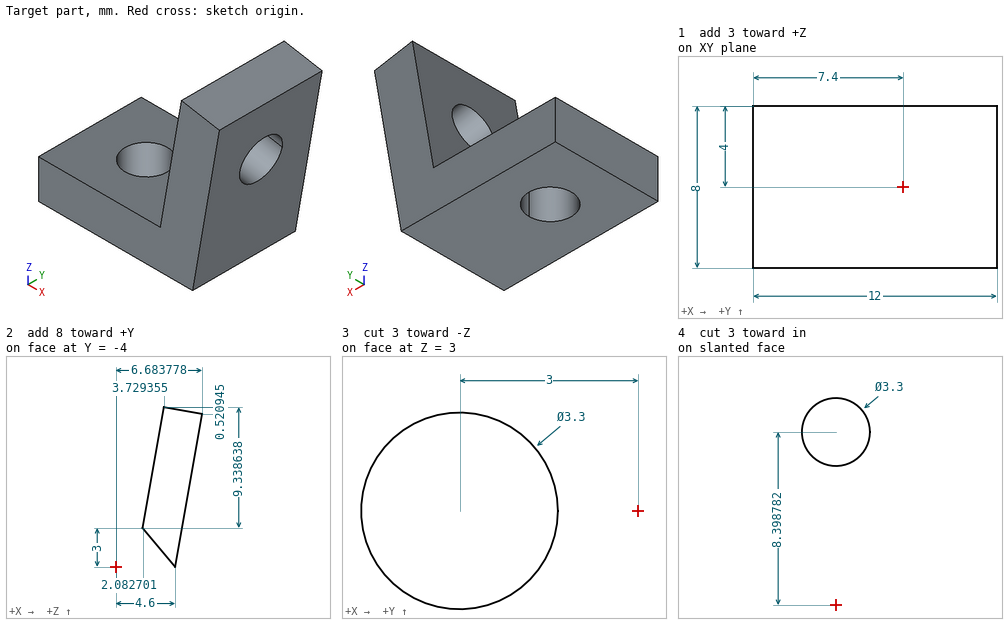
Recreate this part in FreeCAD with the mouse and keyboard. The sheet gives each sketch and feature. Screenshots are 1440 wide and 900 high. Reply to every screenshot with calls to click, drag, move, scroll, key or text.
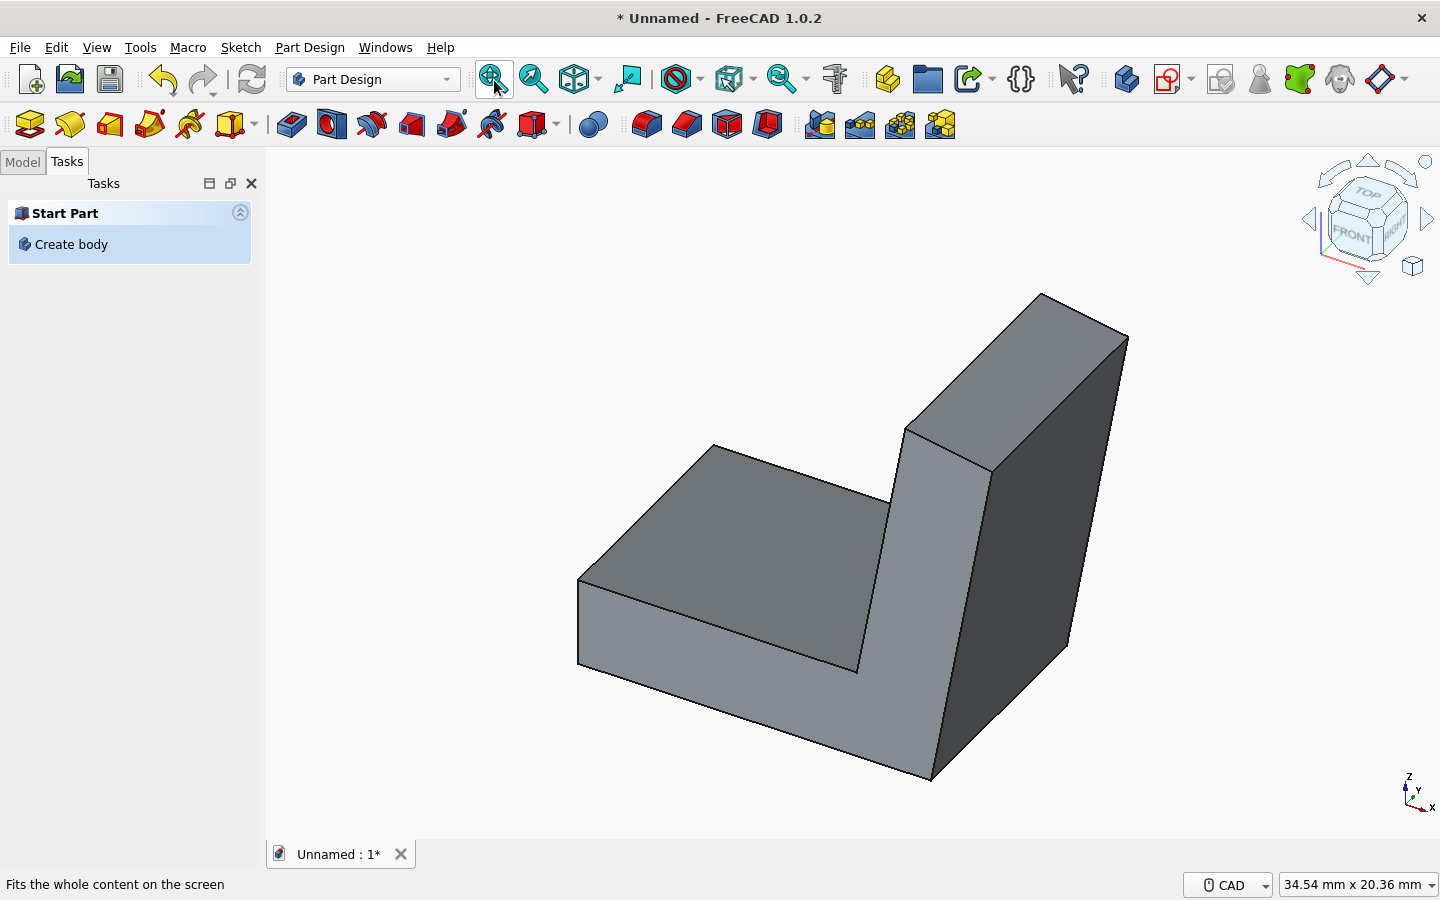
click(785, 558)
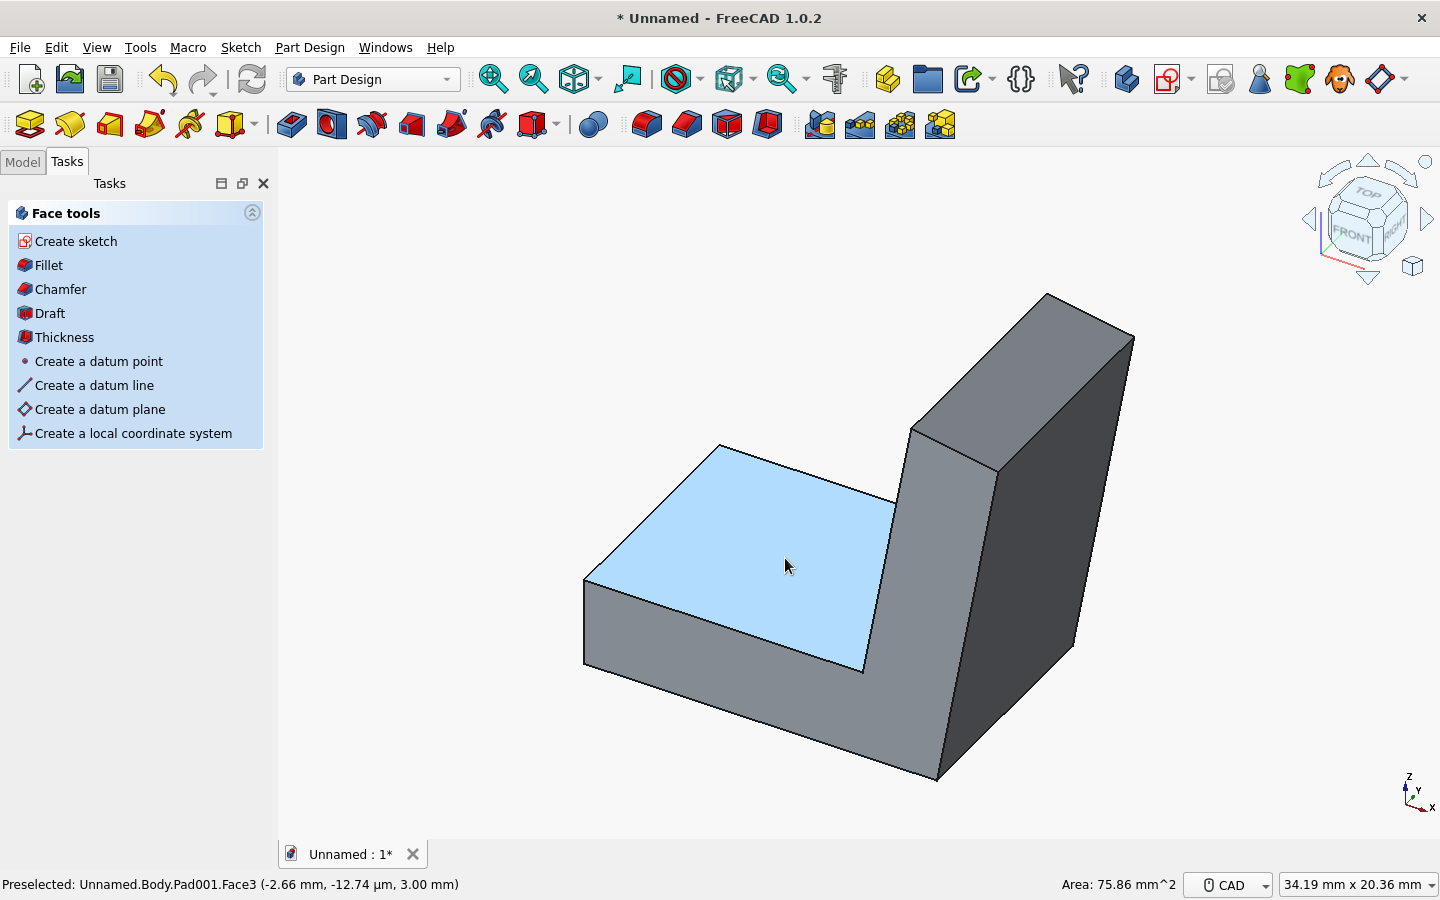
click(1168, 80)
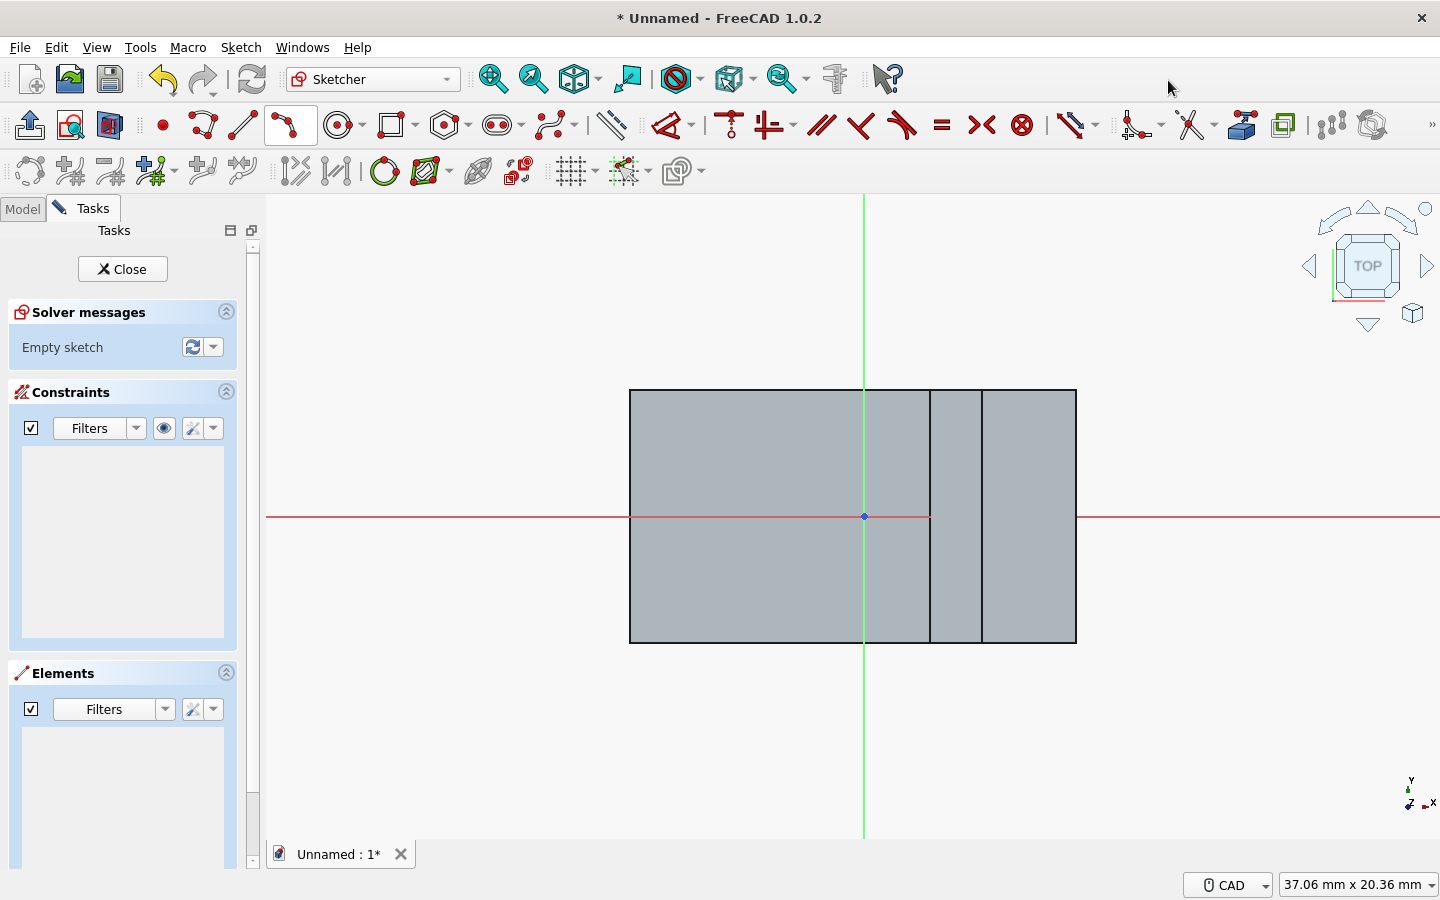
key(q)
key(s)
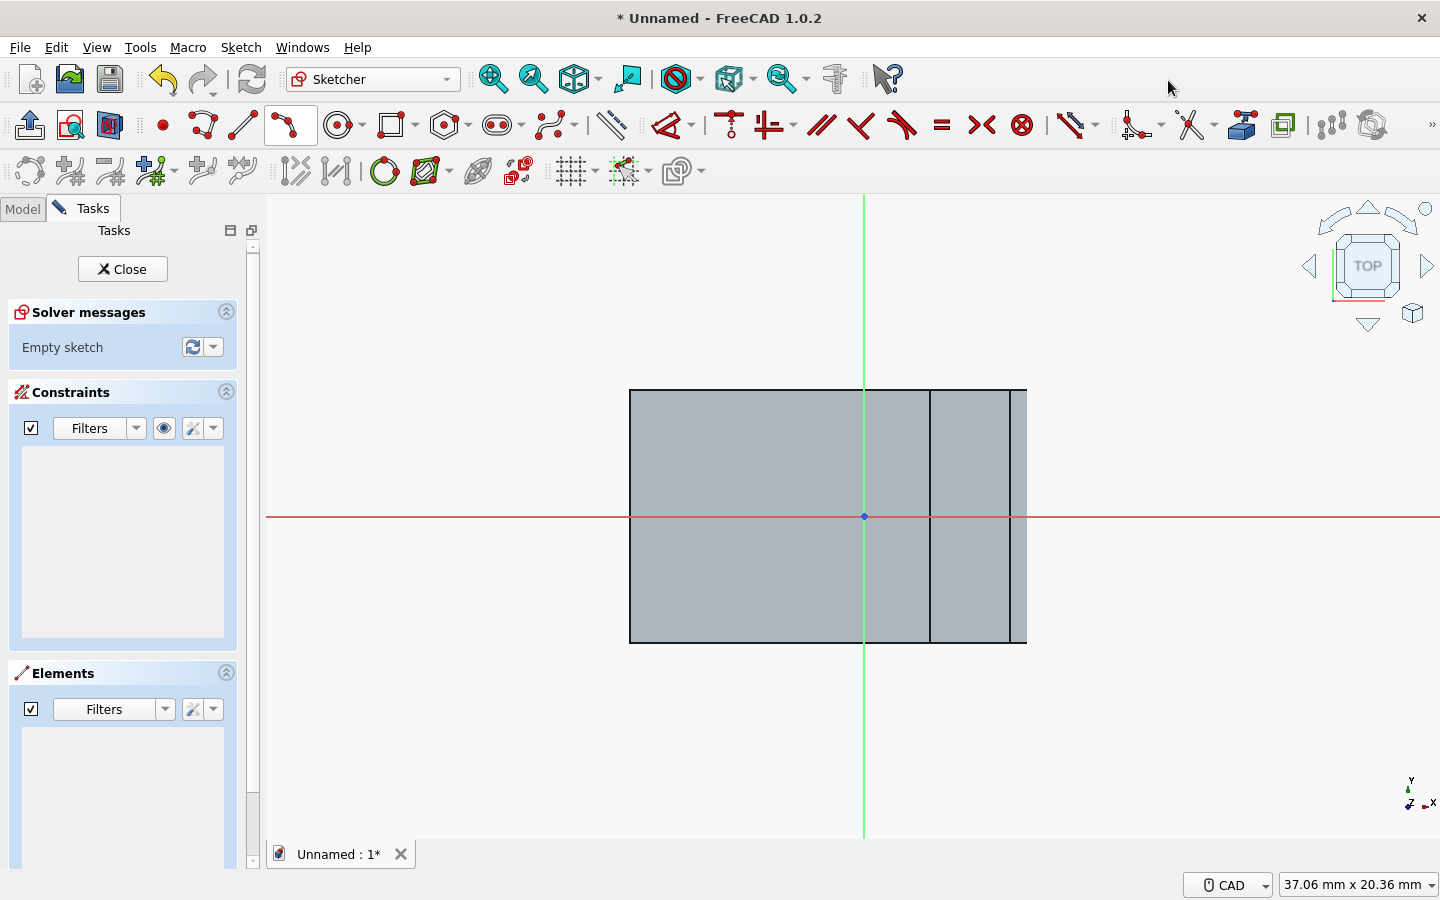
scroll(793, 516, up, 7)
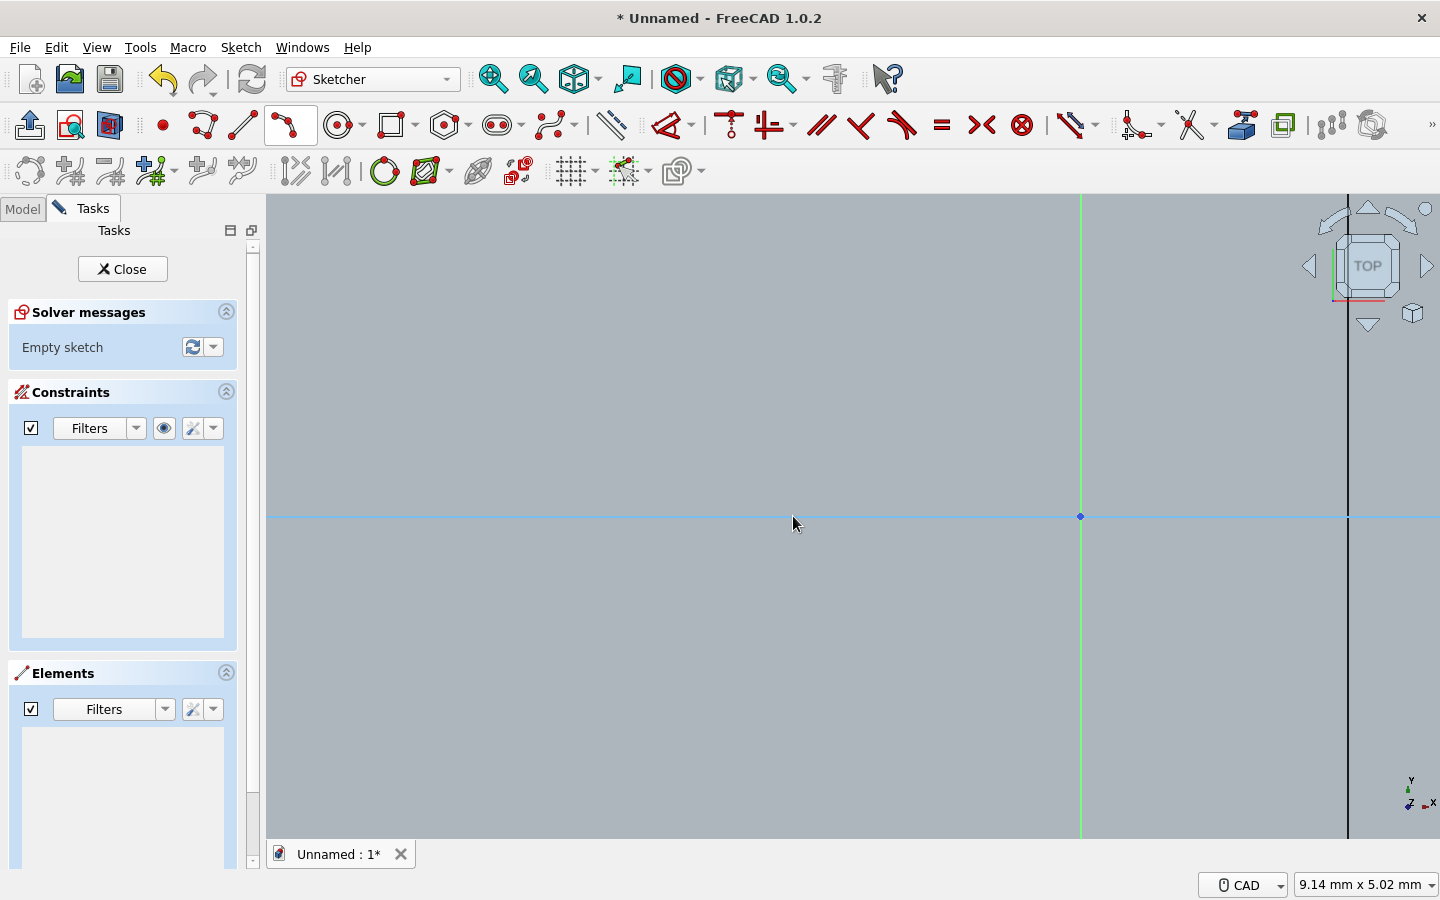
key(g)
key(c)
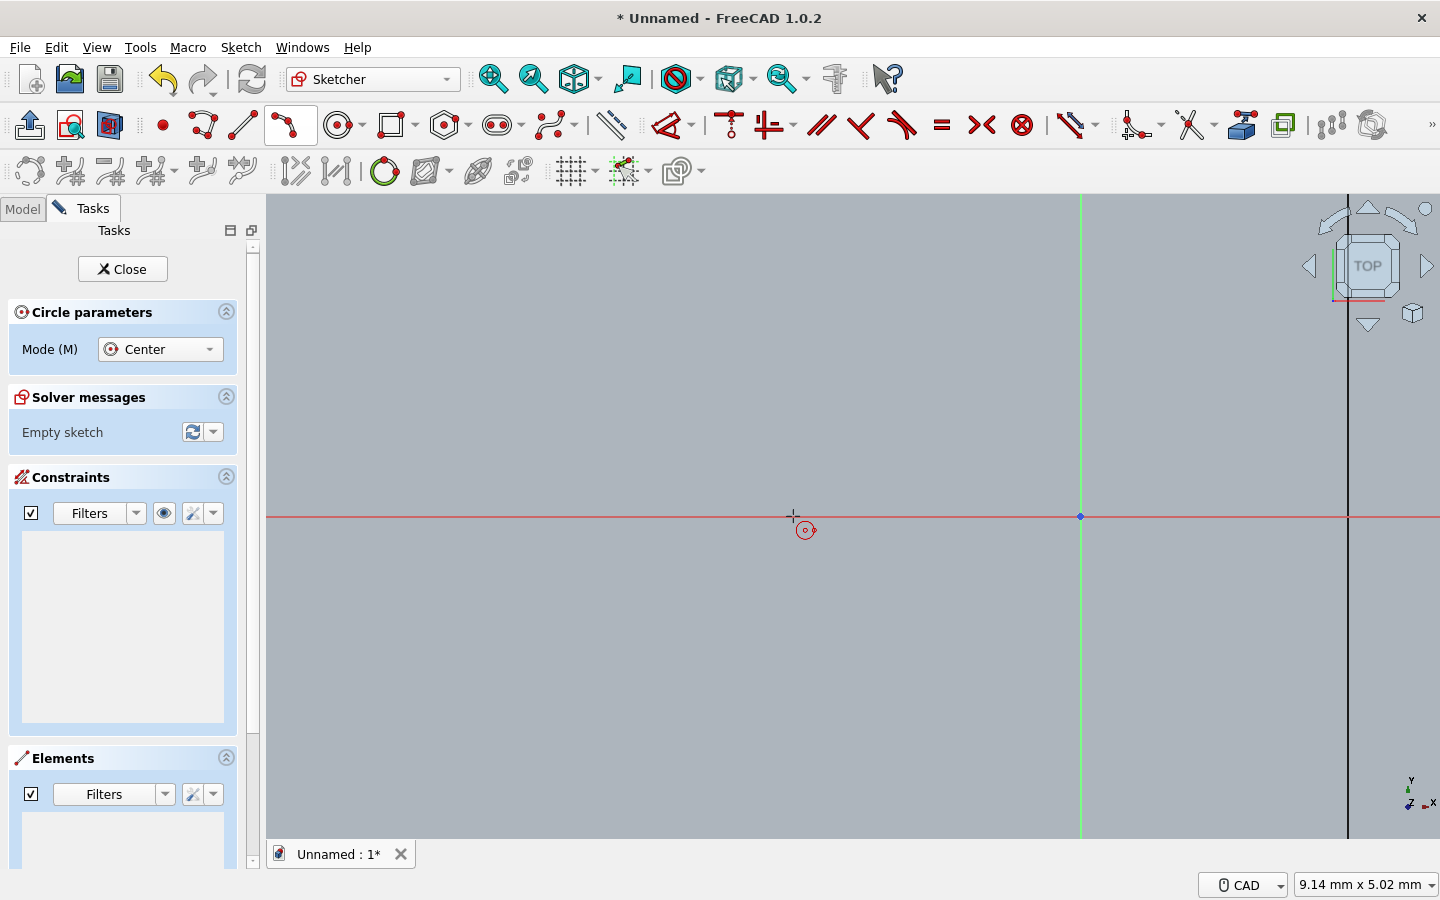
click(696, 516)
click(845, 367)
key(Escape)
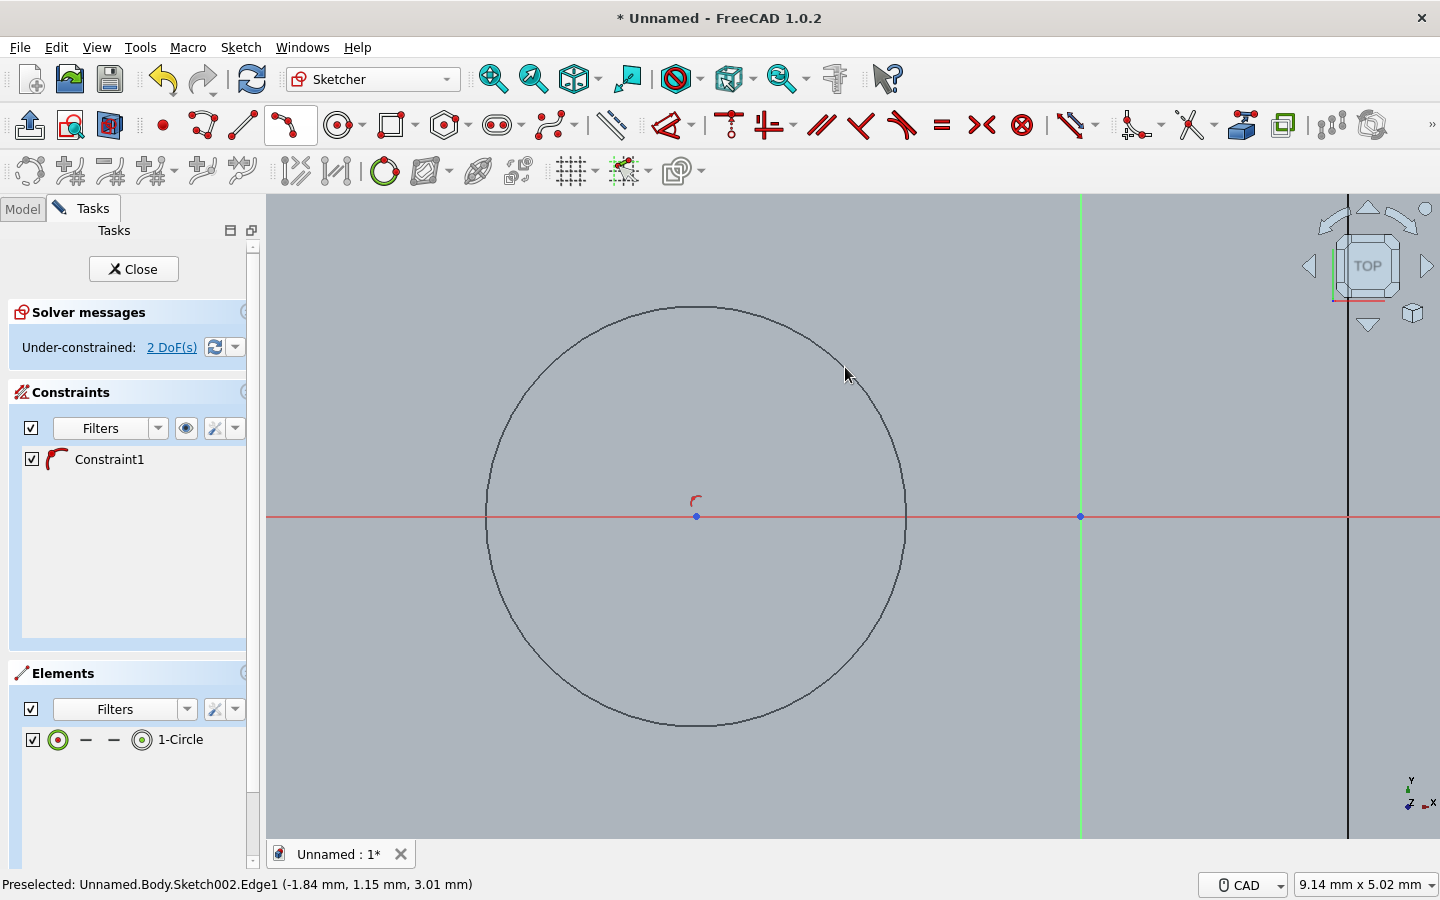
key(d)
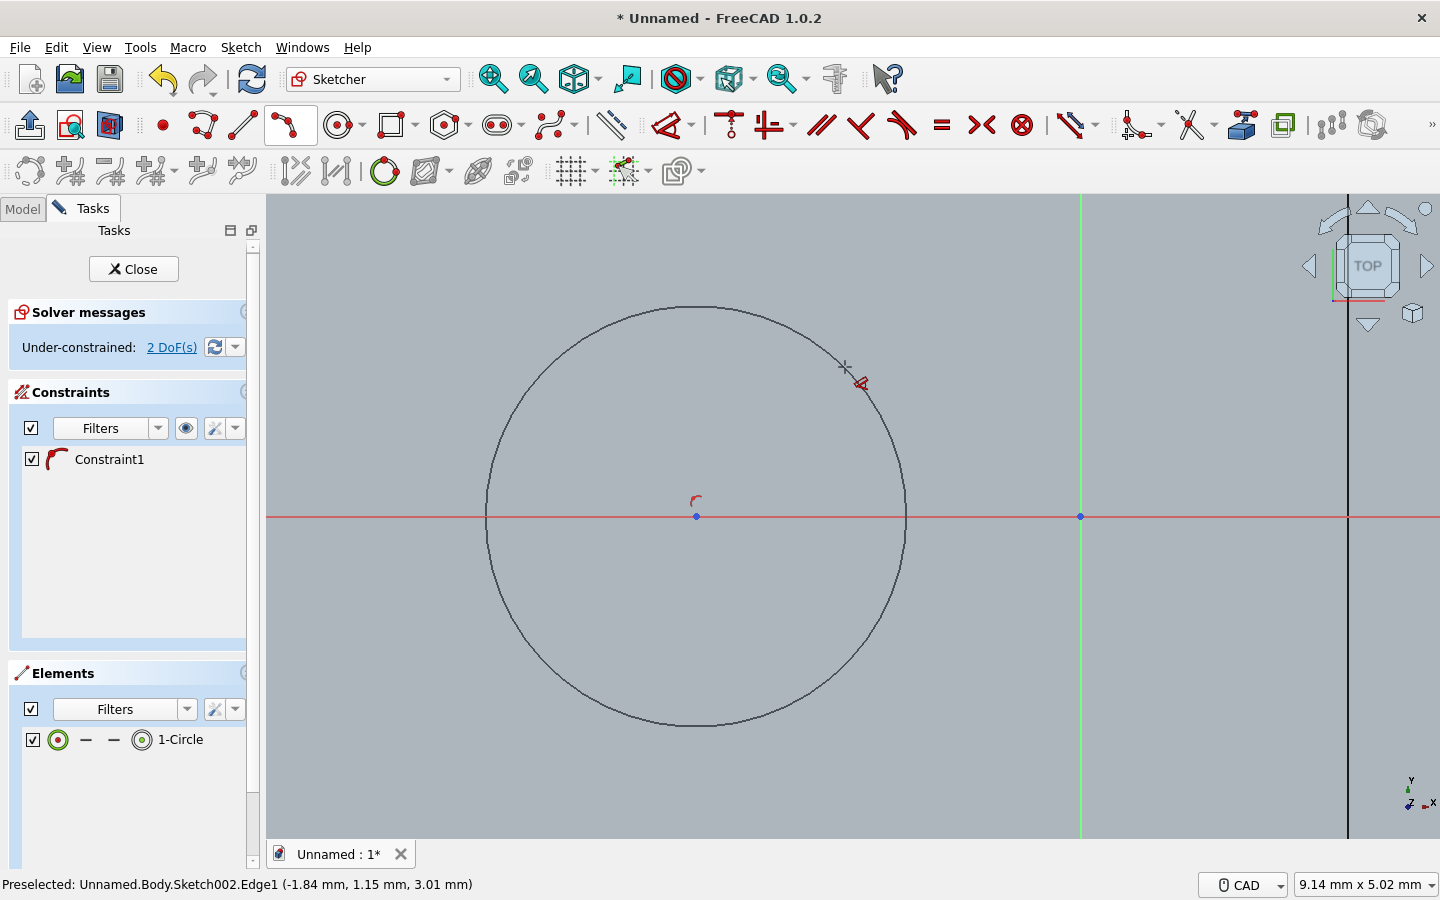
click(844, 367)
click(867, 344)